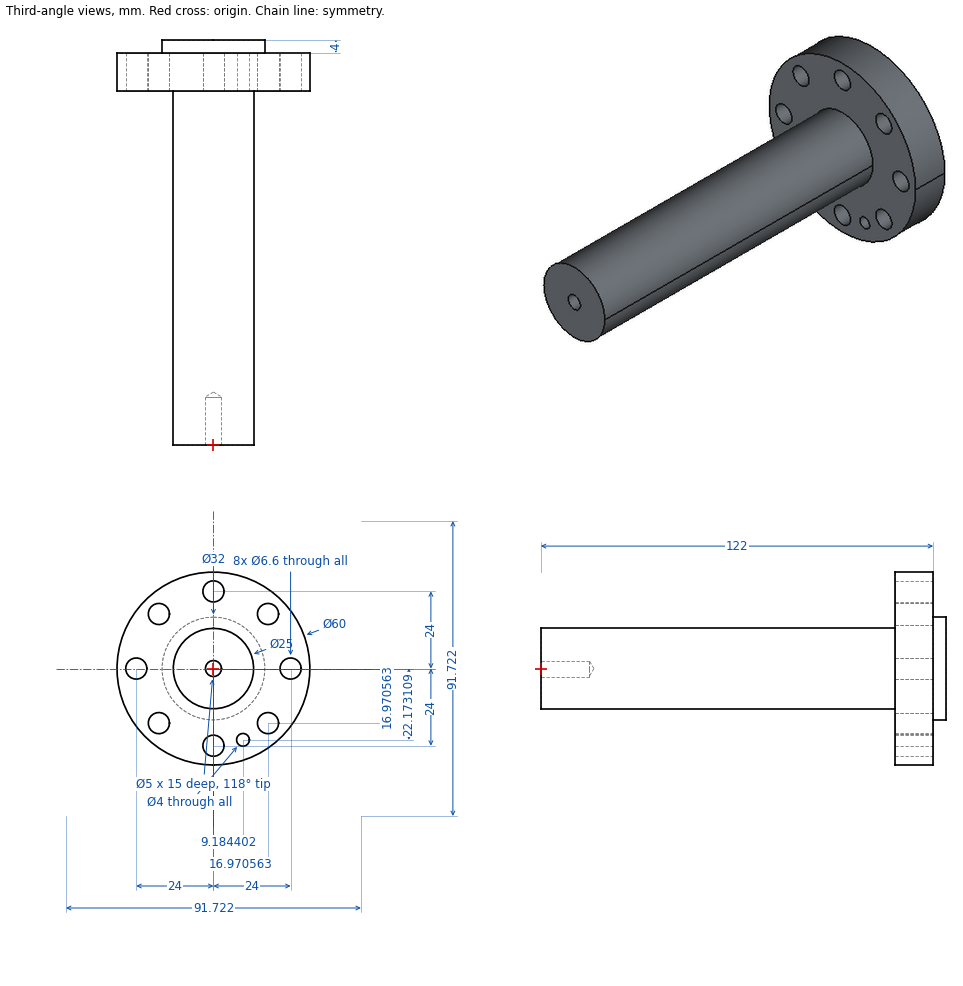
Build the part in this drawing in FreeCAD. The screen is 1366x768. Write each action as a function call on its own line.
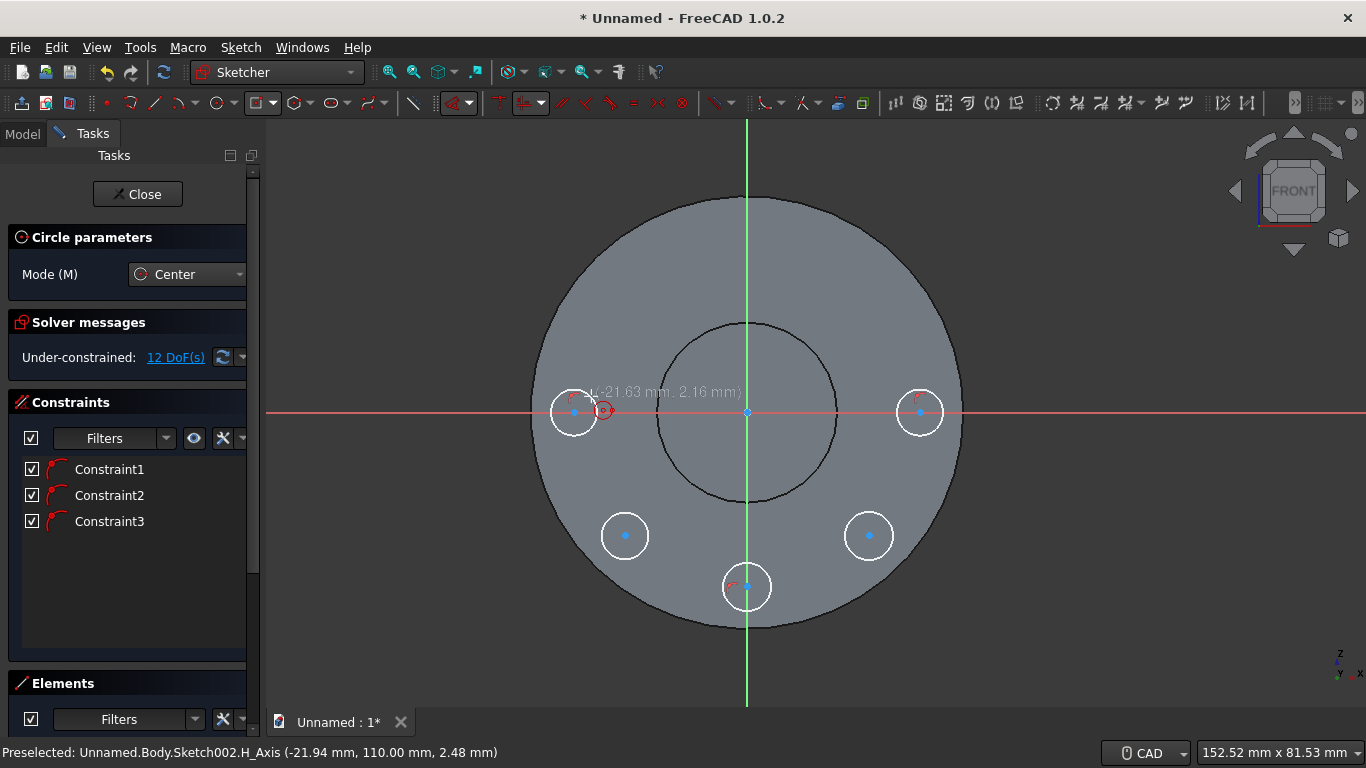
click(625, 290)
click(641, 273)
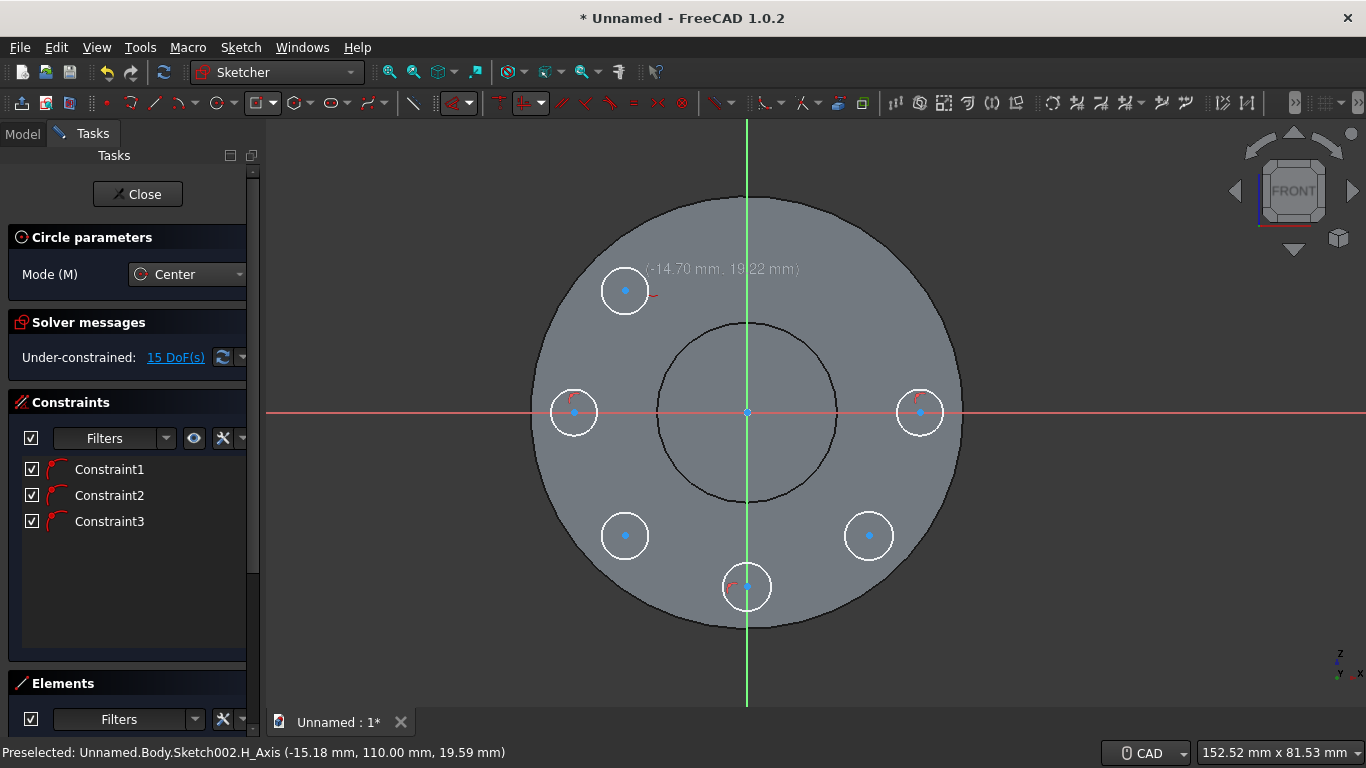
click(747, 239)
click(764, 223)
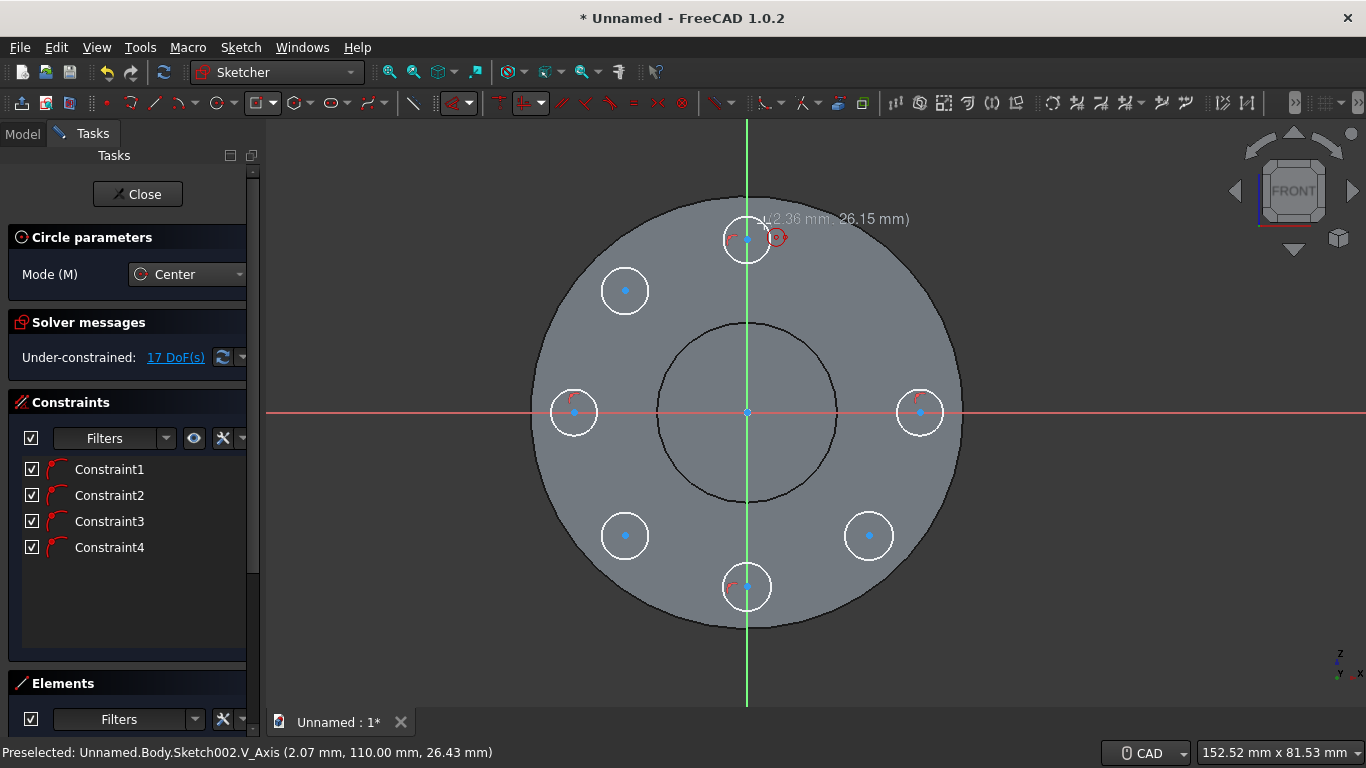
click(869, 290)
click(886, 273)
key(Escape)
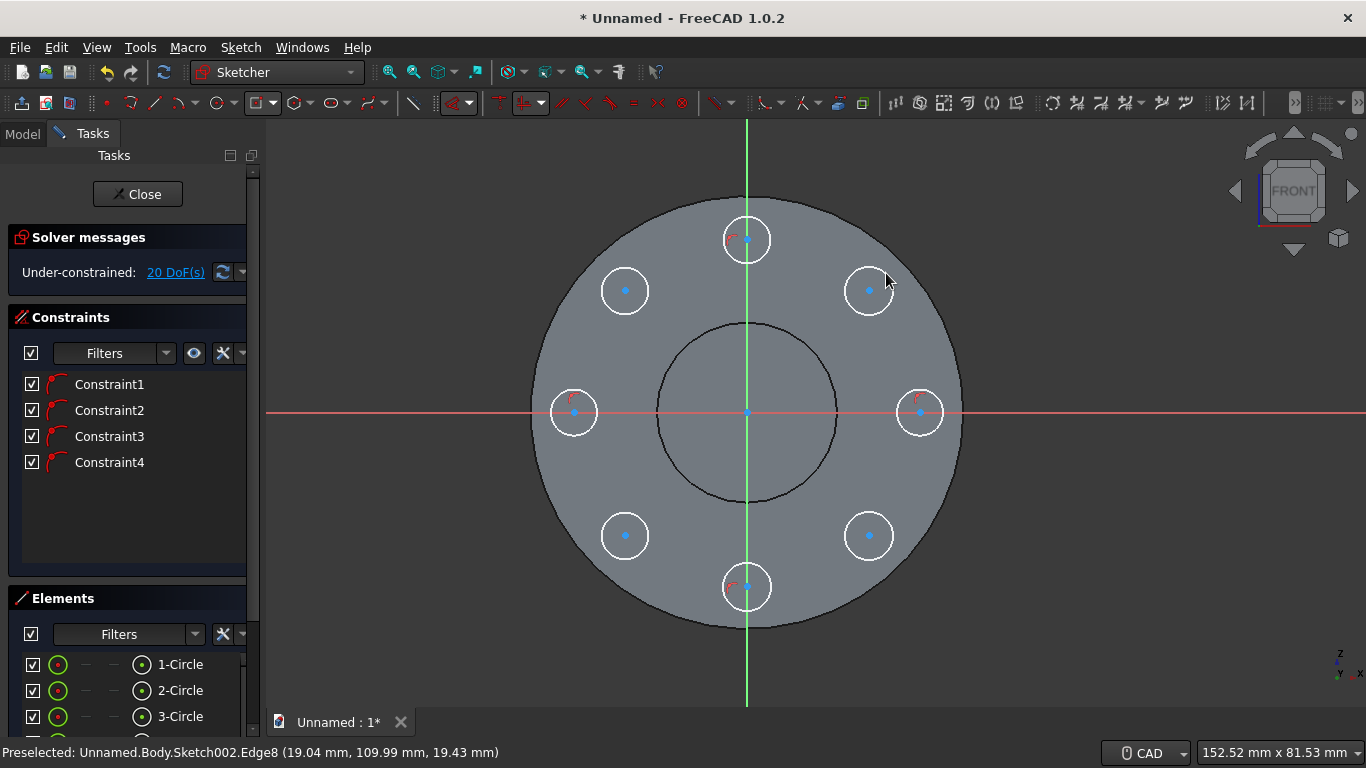
click(936, 396)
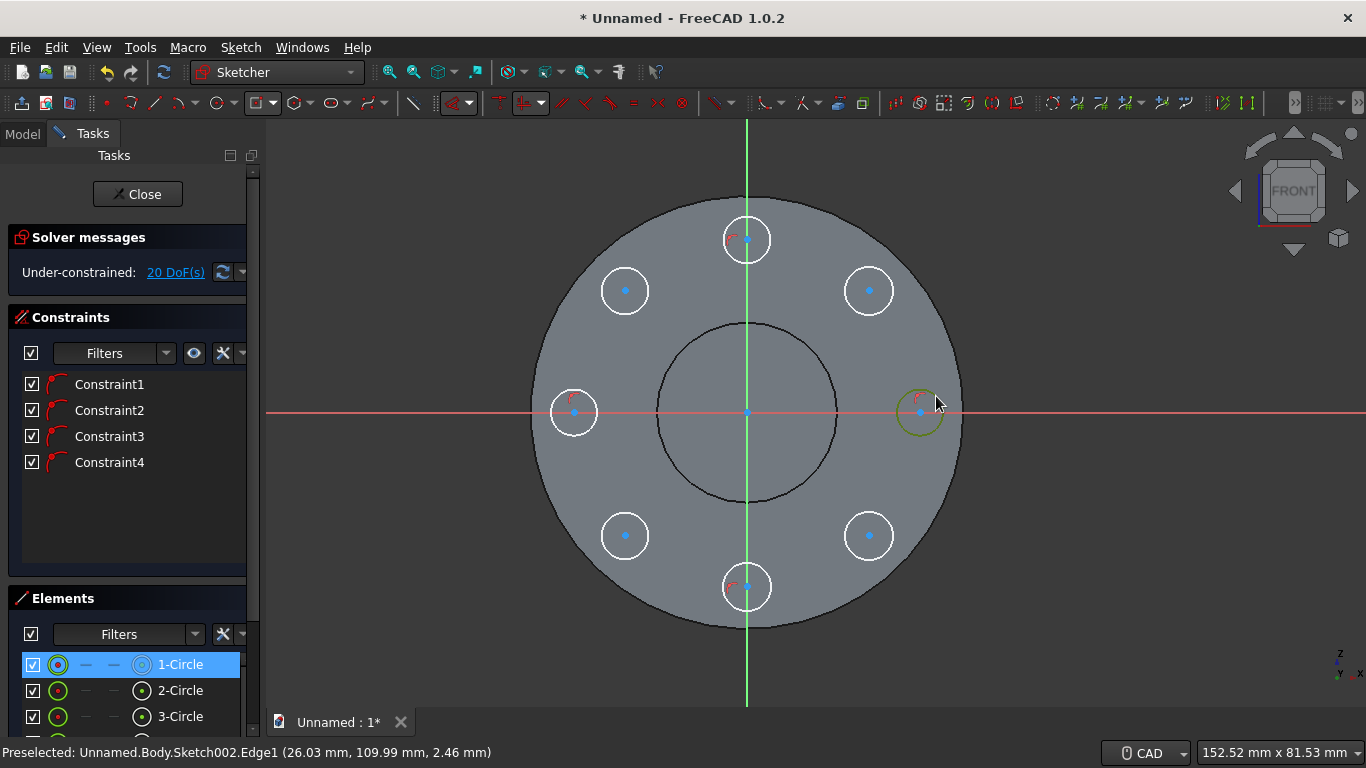
click(886, 519)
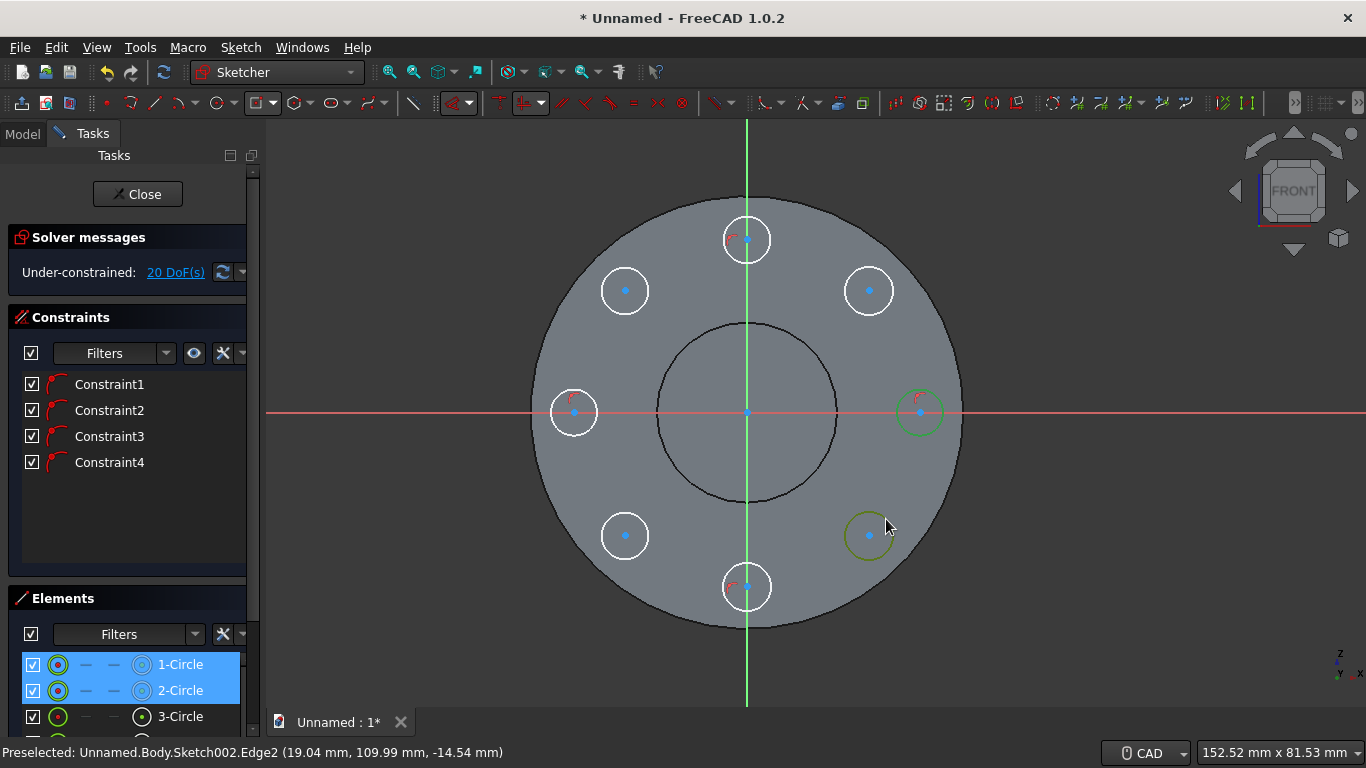
click(764, 570)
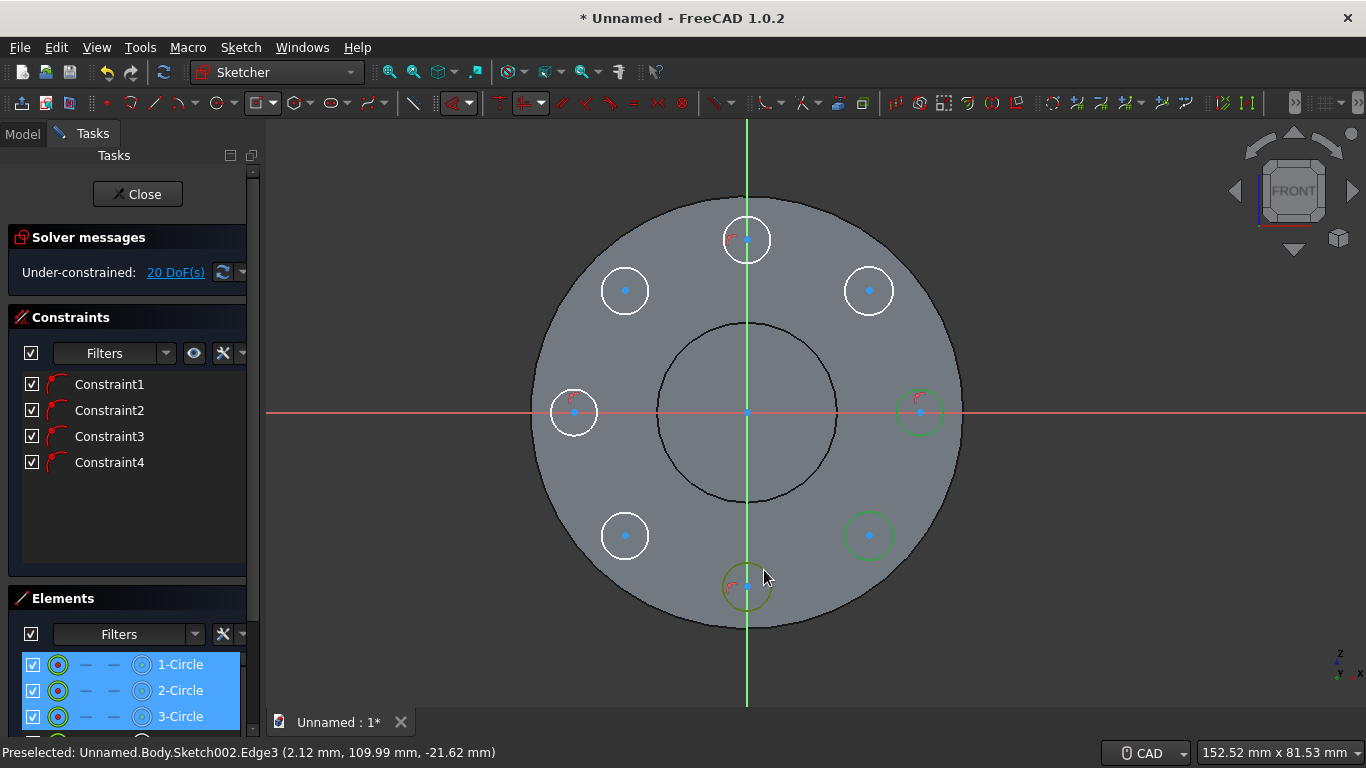
click(641, 519)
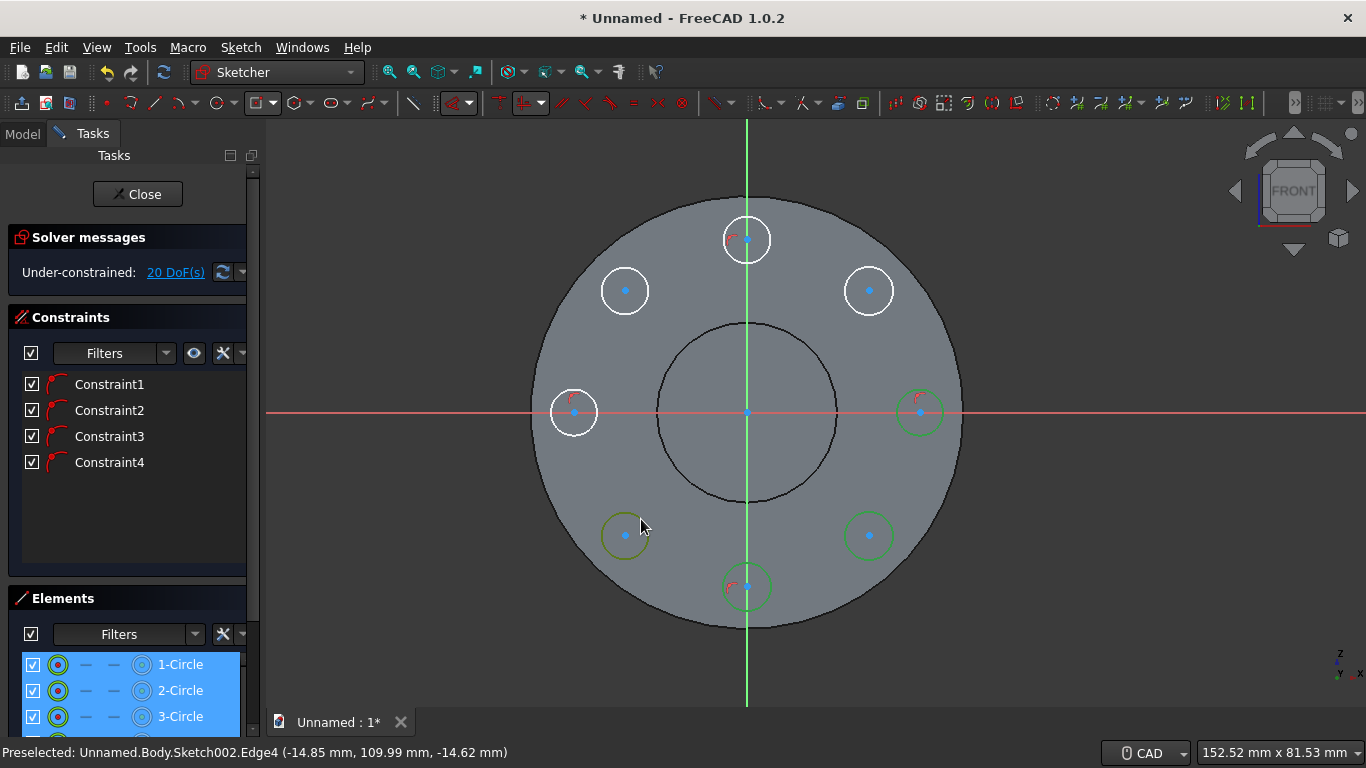
click(590, 396)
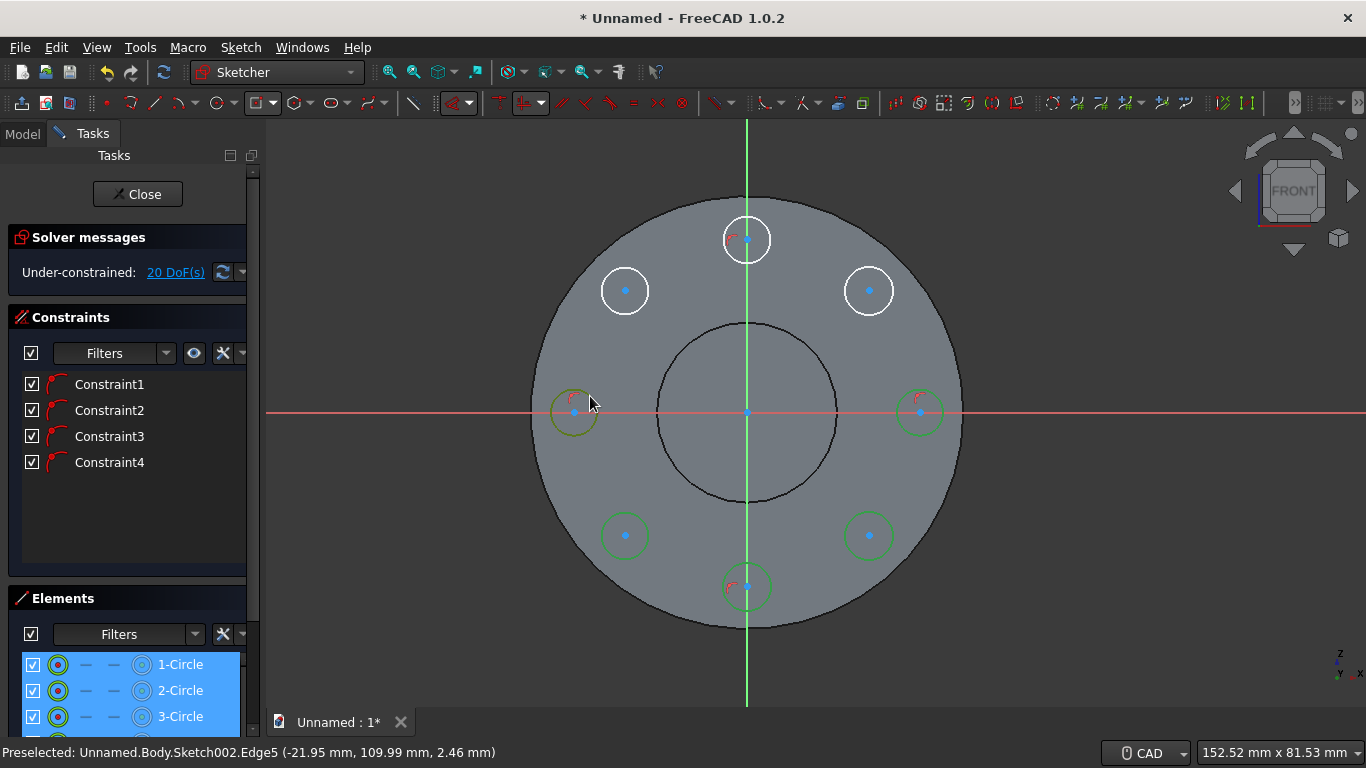
click(641, 274)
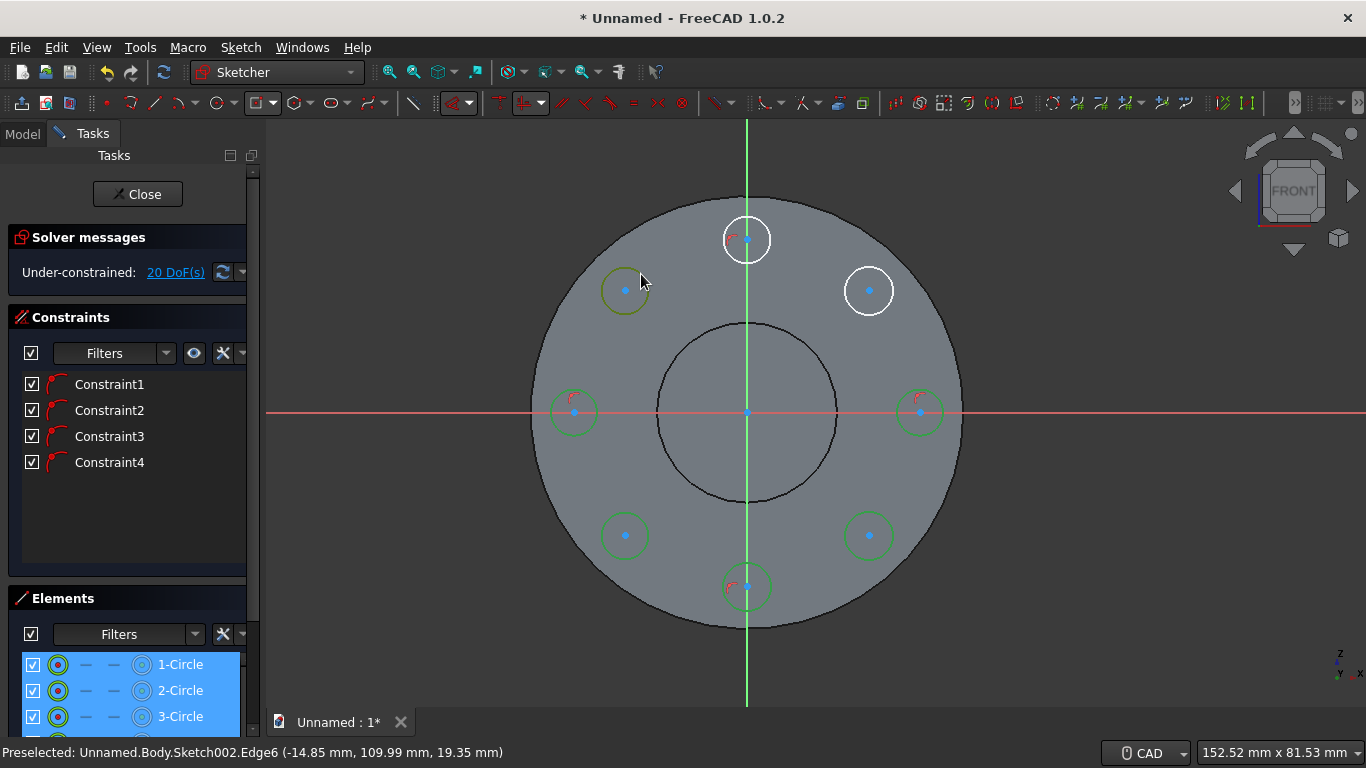
click(763, 223)